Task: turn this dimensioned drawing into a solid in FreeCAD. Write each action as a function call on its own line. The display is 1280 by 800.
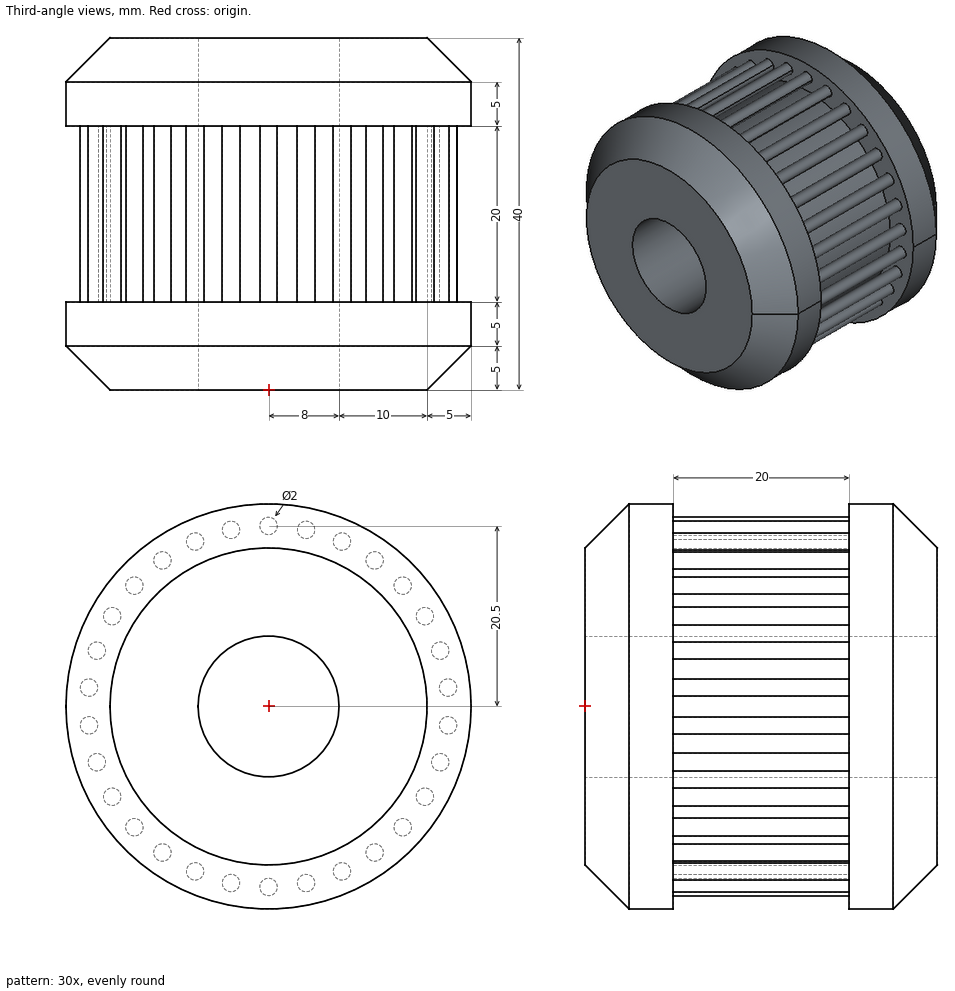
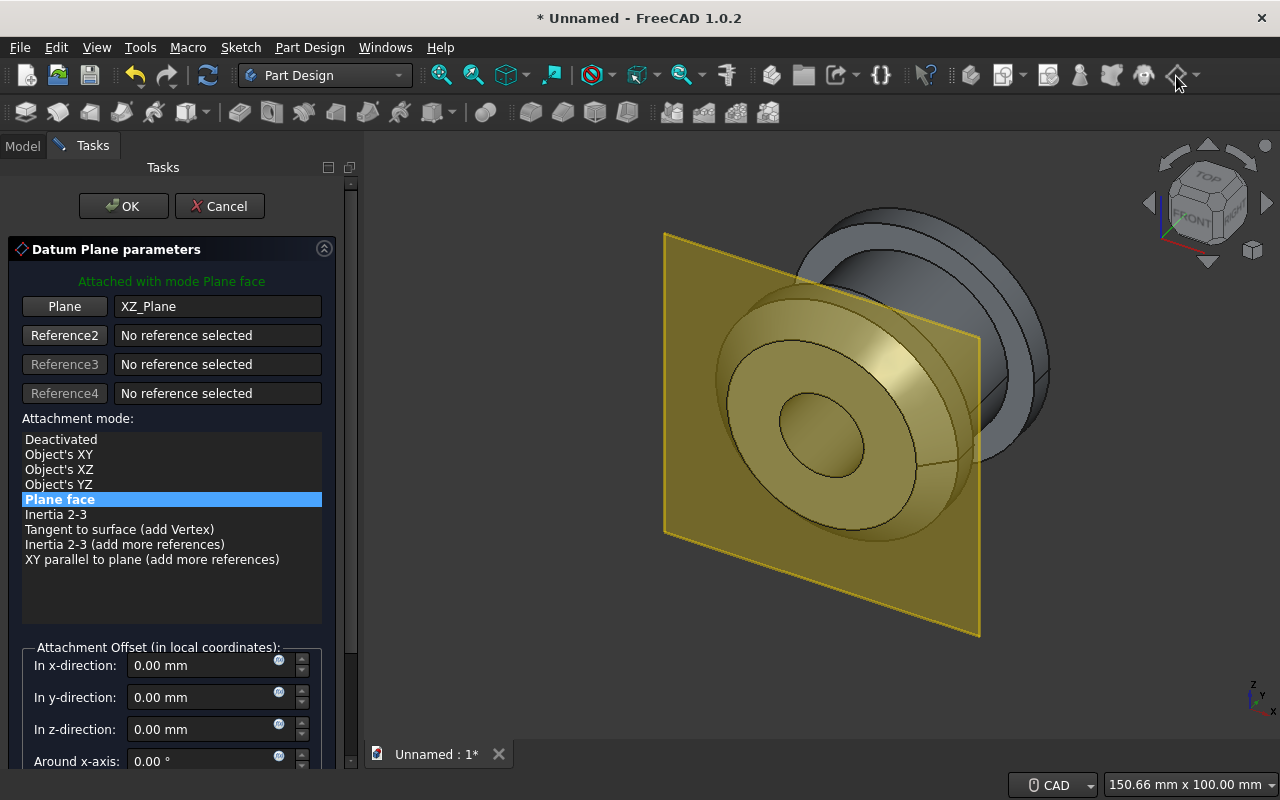
triple_click(210, 729)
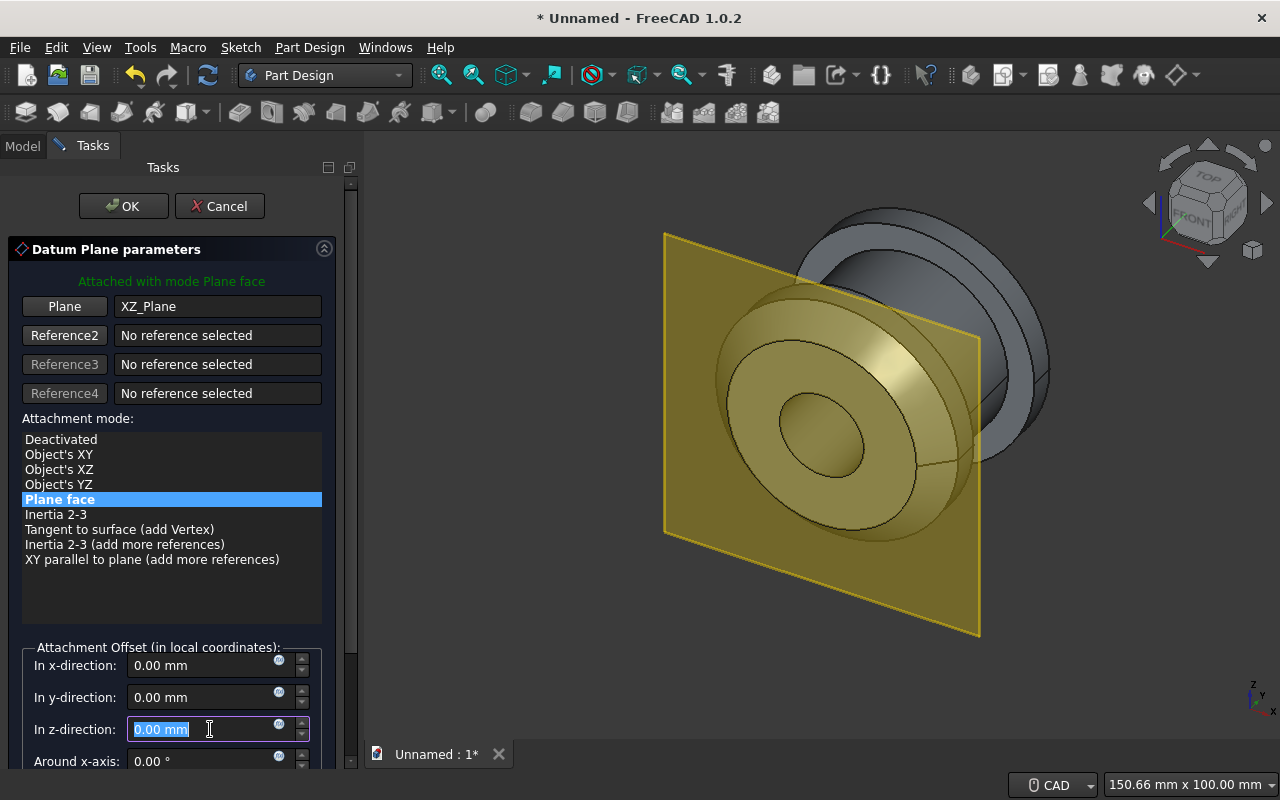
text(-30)
key(Tab)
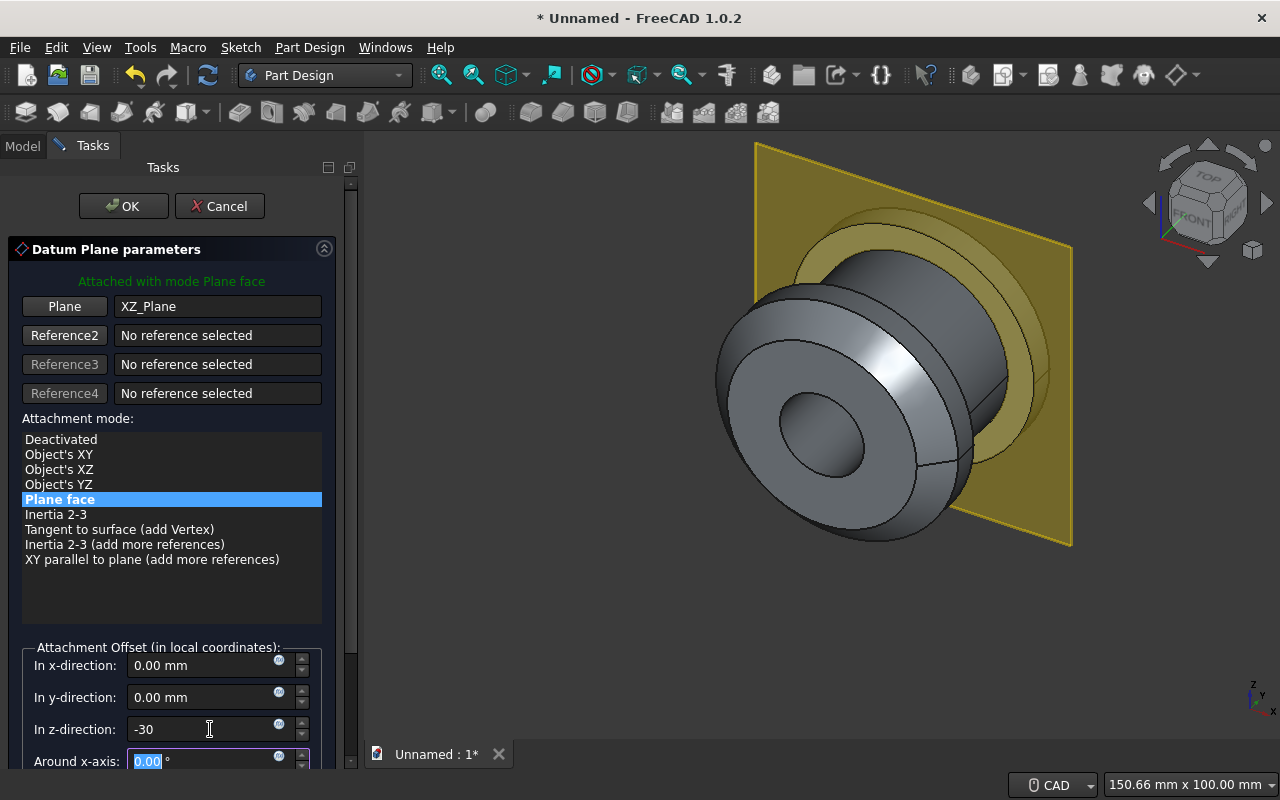
click(124, 206)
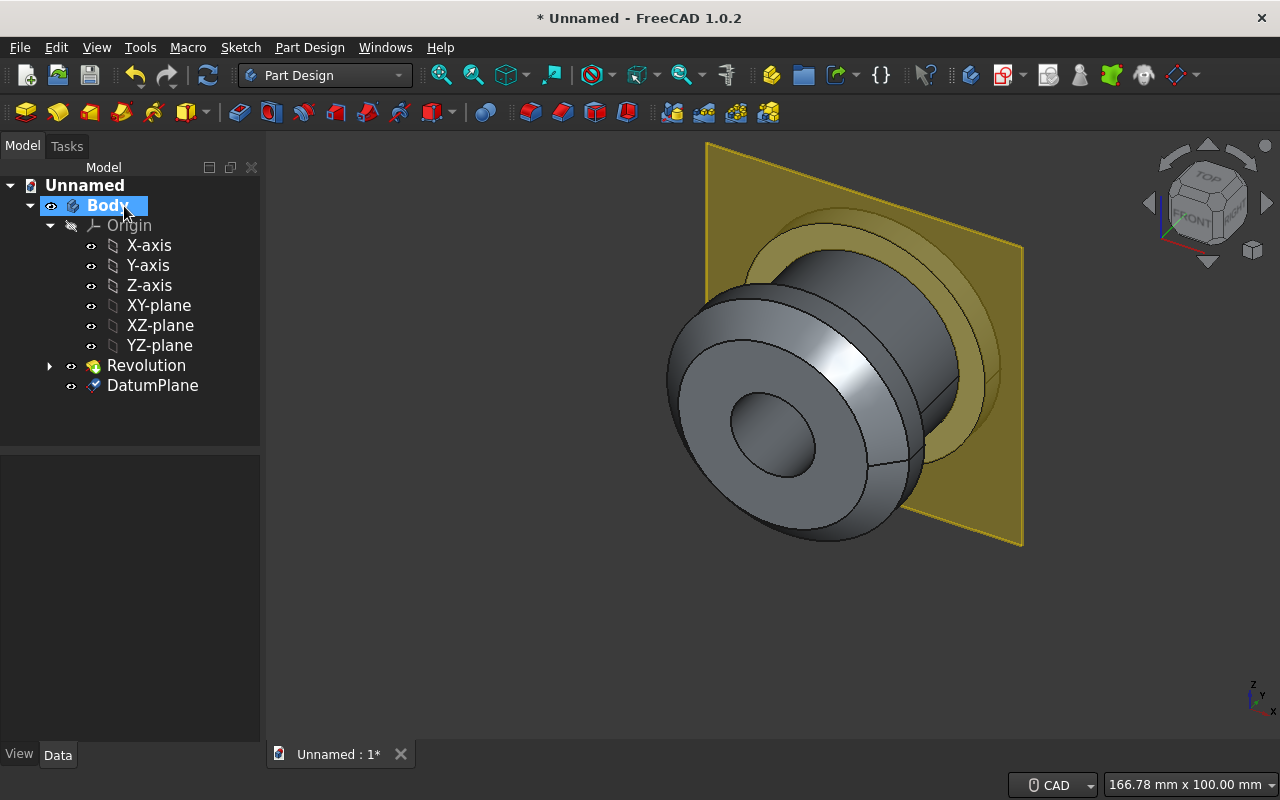
click(116, 386)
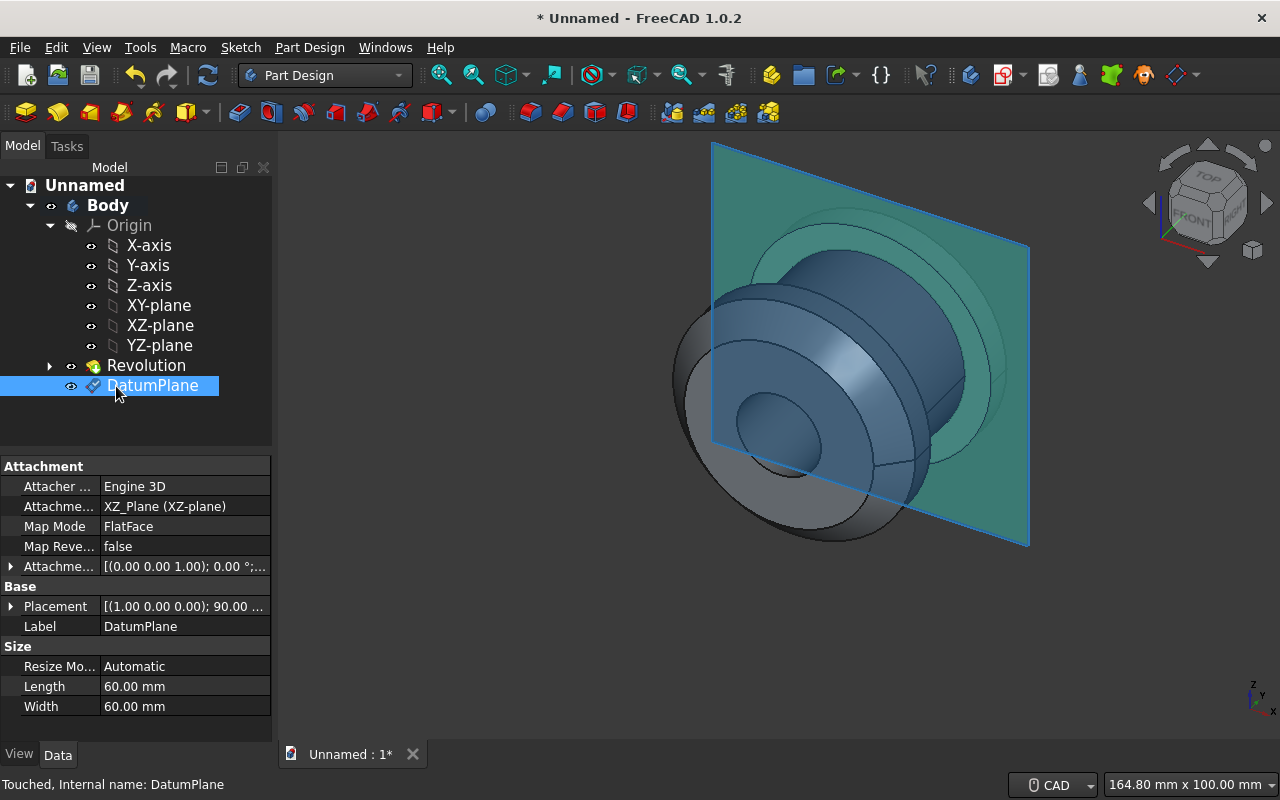
click(1004, 76)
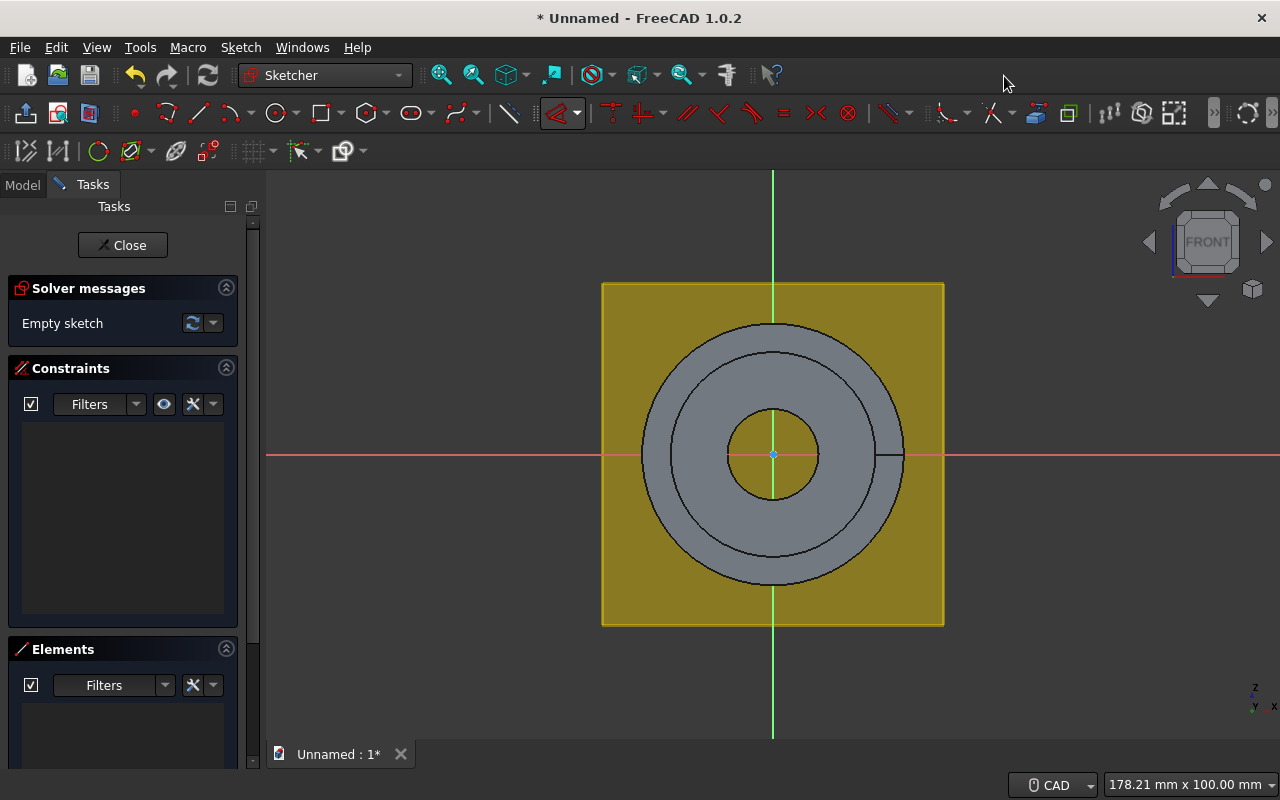
key(q)
key(s)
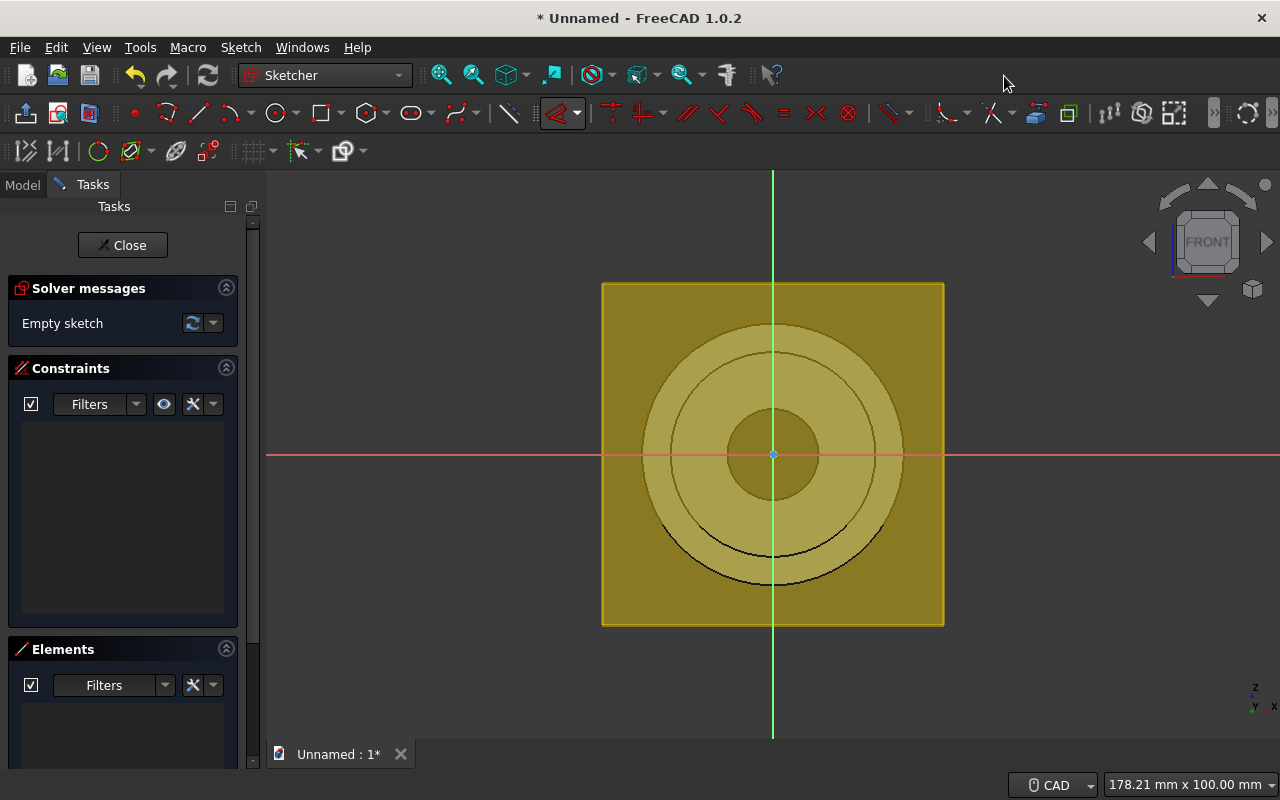
scroll(777, 332, up, 15)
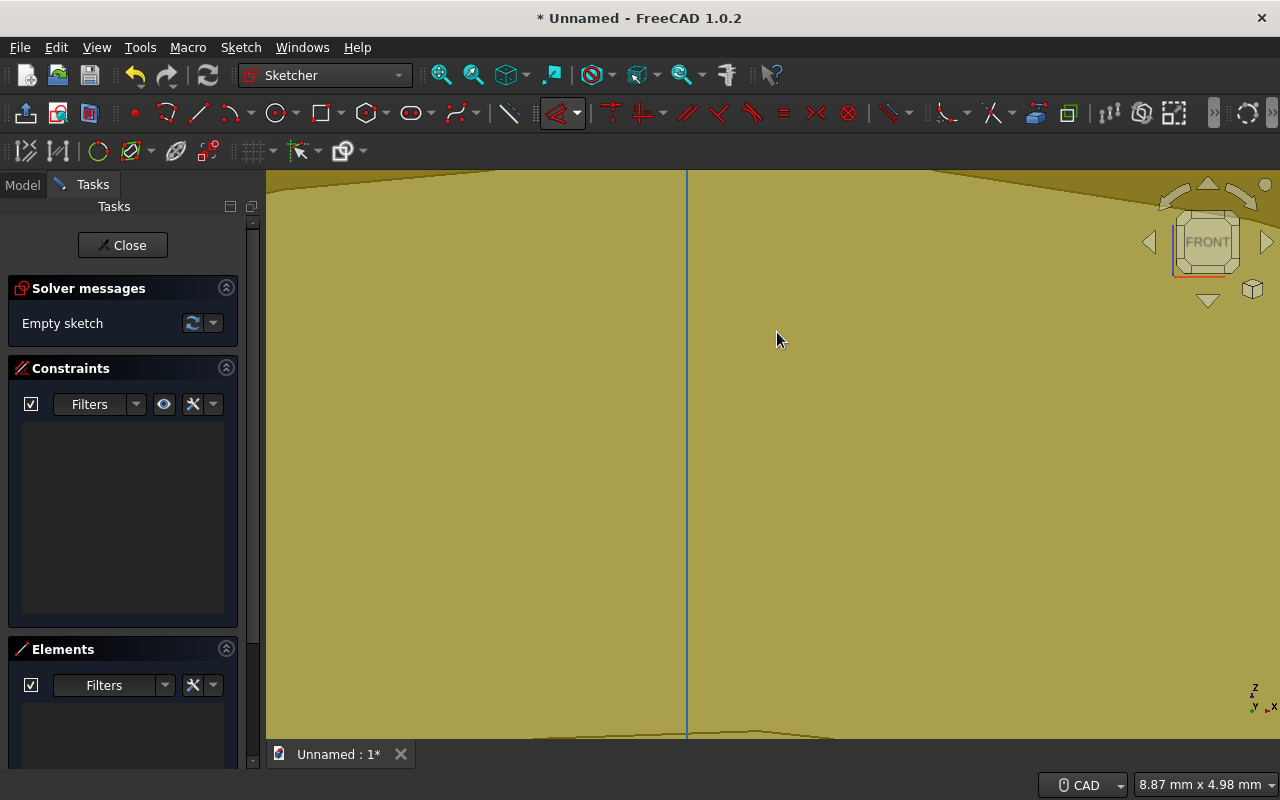
scroll(652, 423, up, 2)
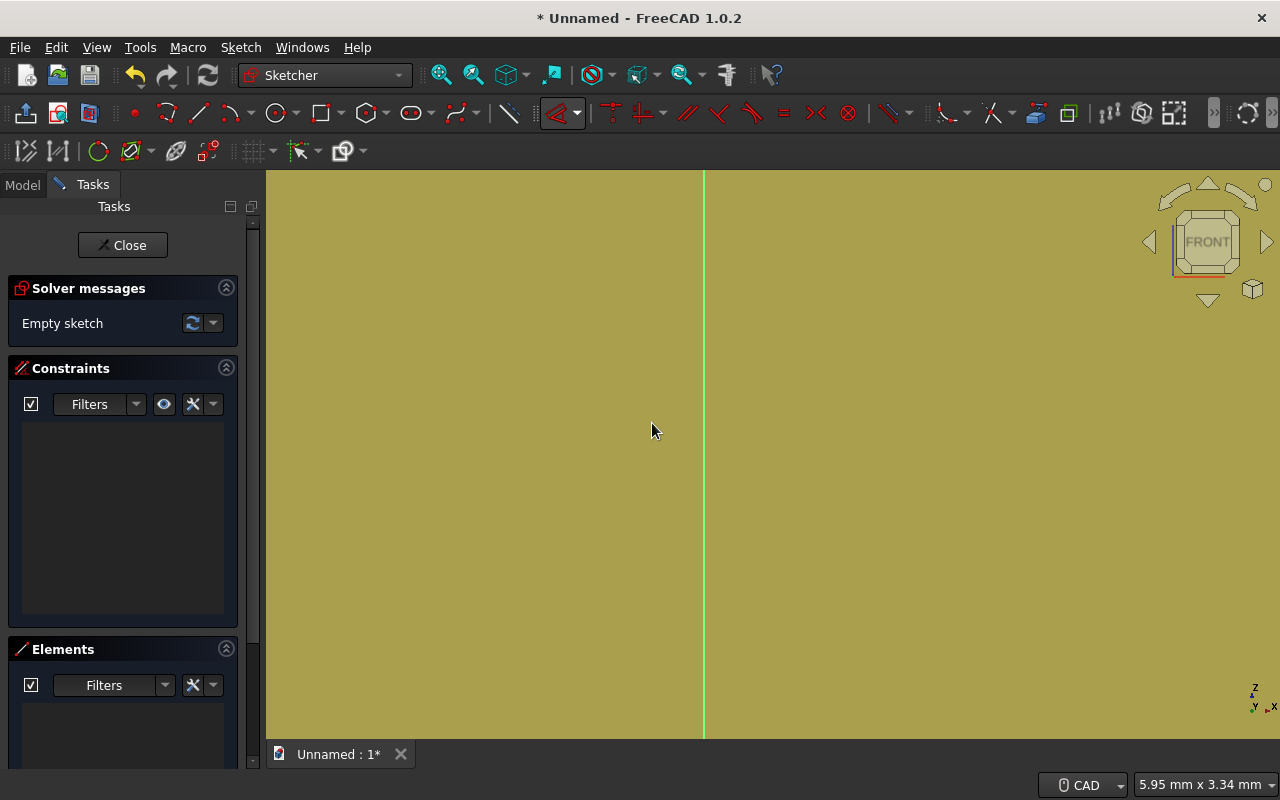
key(g)
key(c)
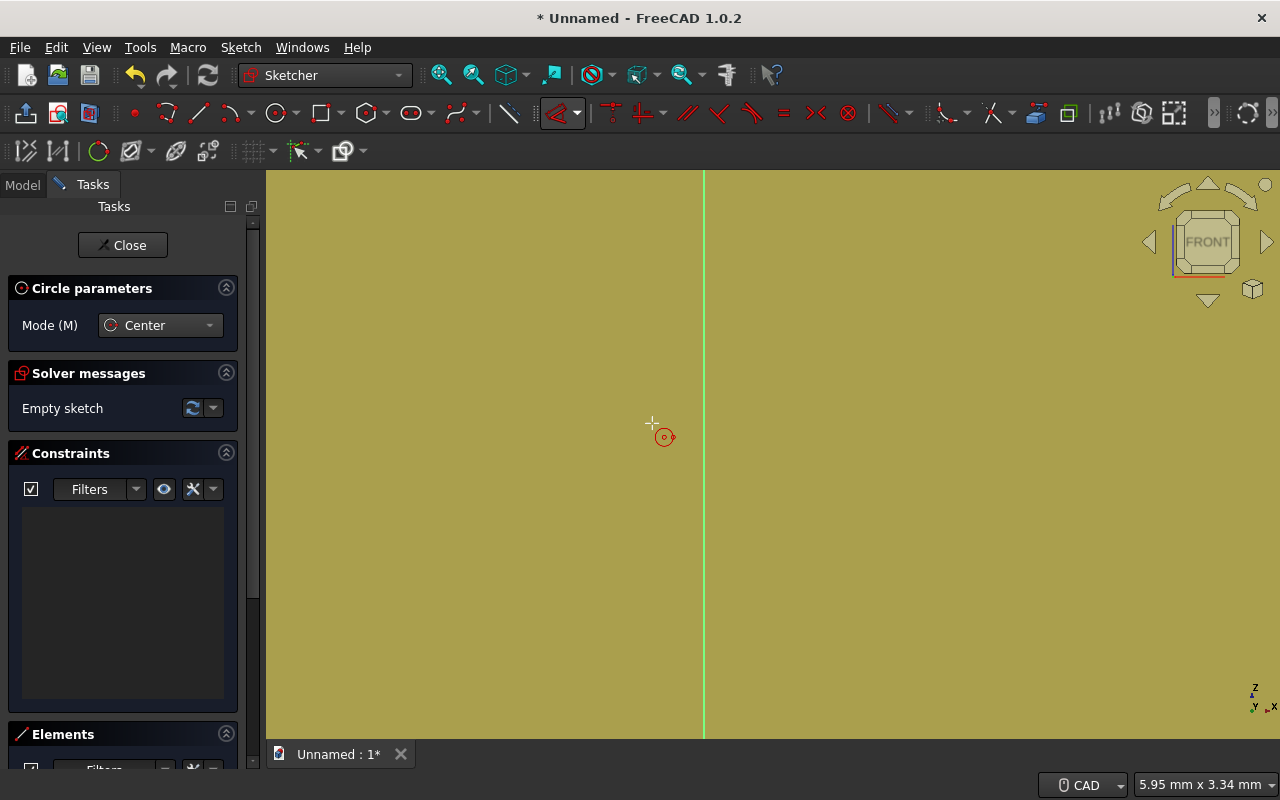
click(704, 454)
click(825, 334)
key(Escape)